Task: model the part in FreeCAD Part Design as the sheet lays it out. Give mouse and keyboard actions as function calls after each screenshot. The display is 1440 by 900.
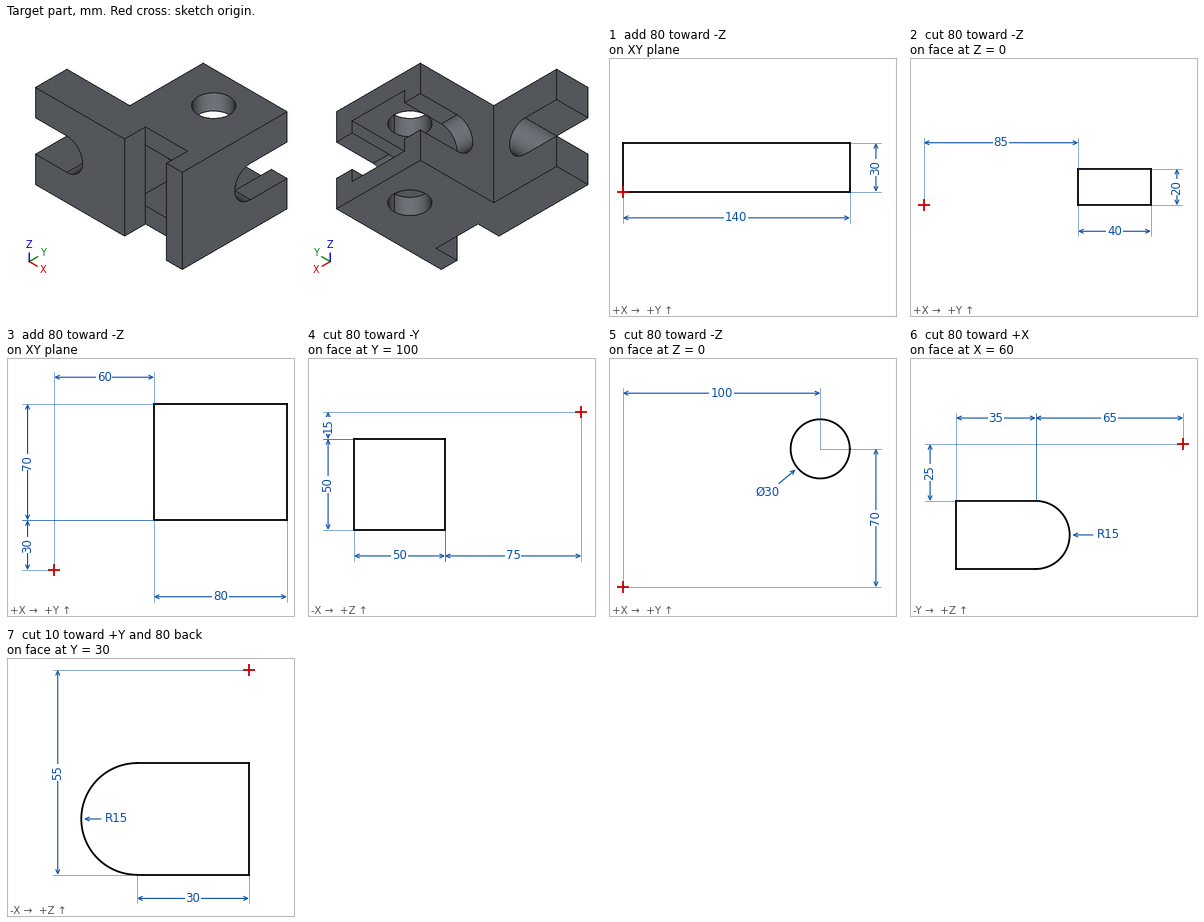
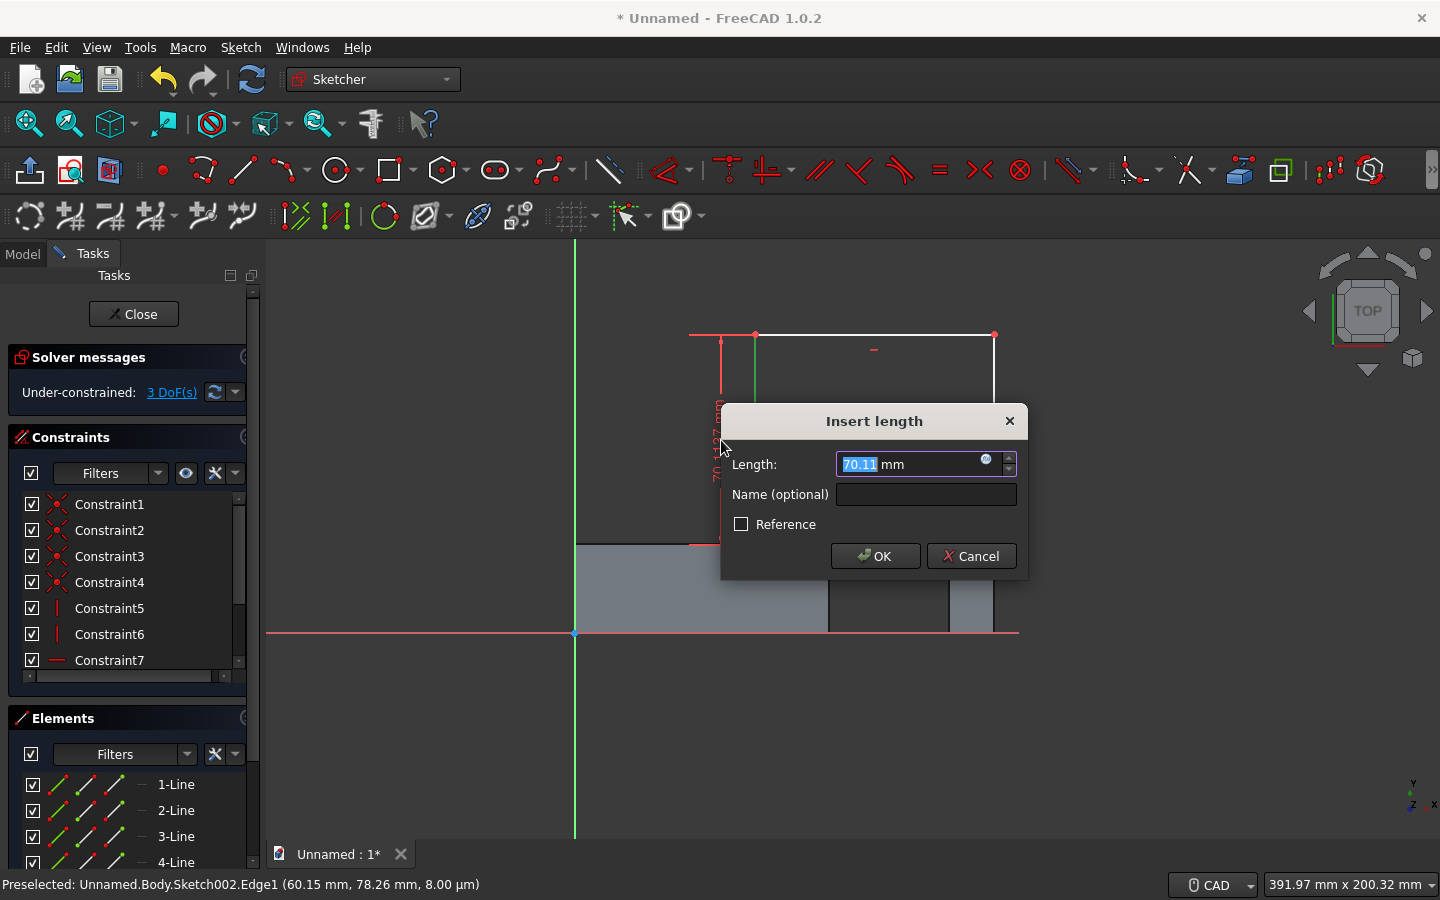
text(70)
key(Return)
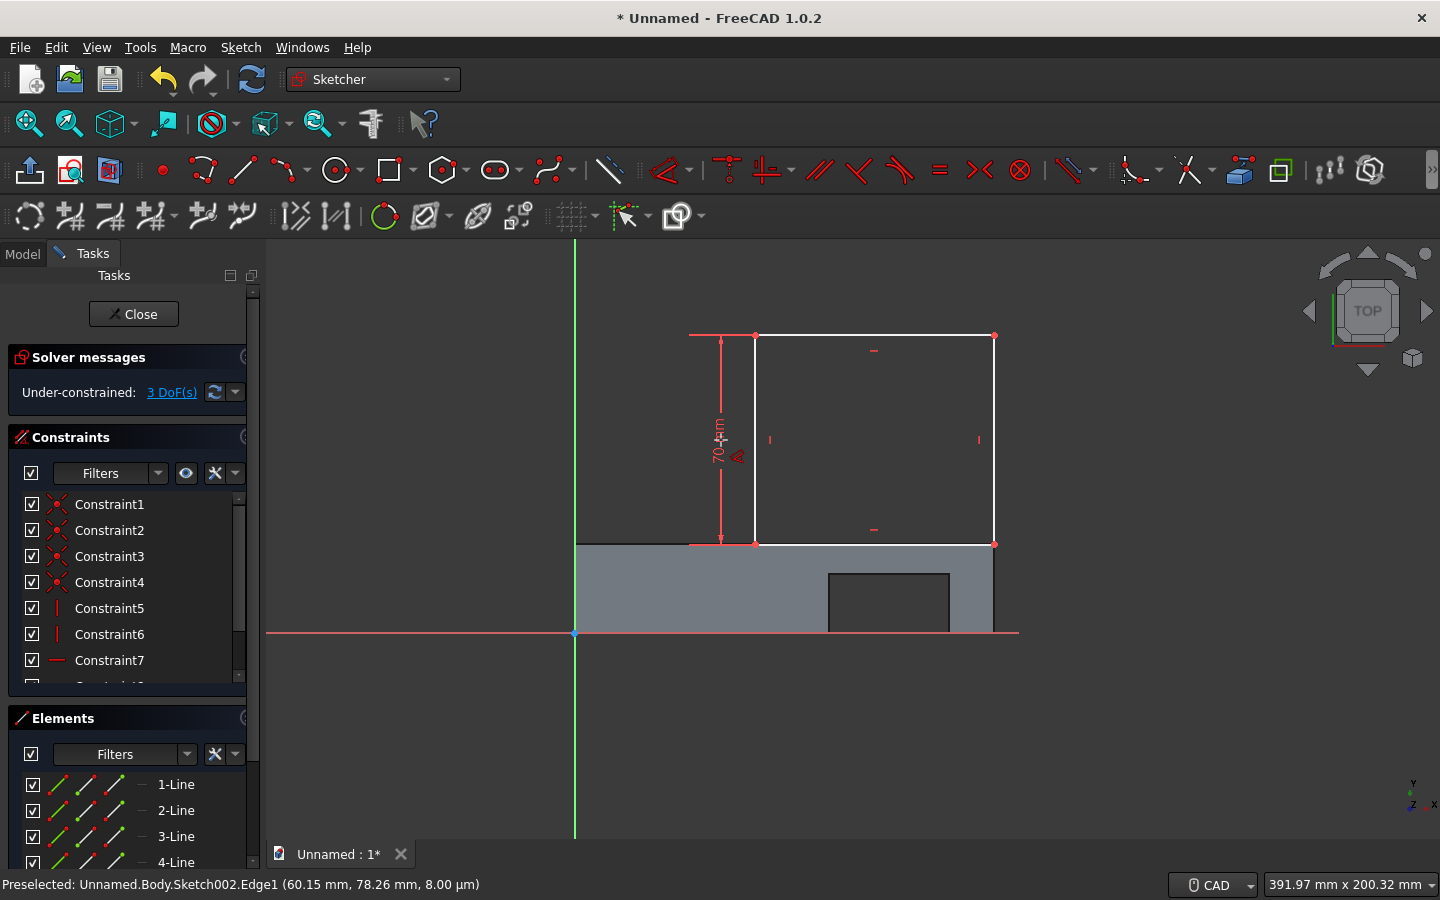
click(827, 545)
click(875, 579)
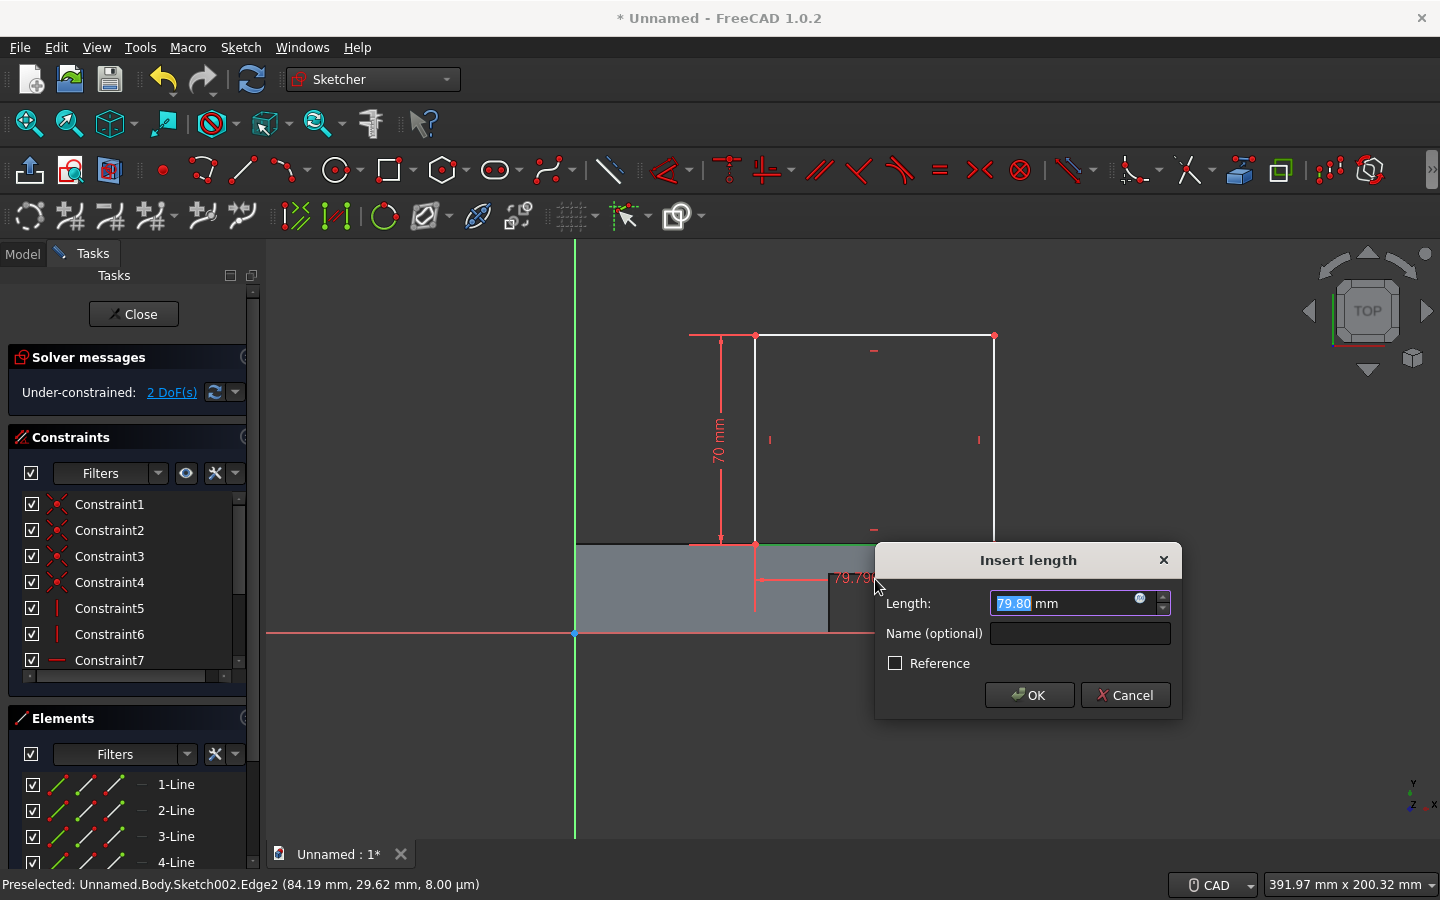
text(80)
key(Return)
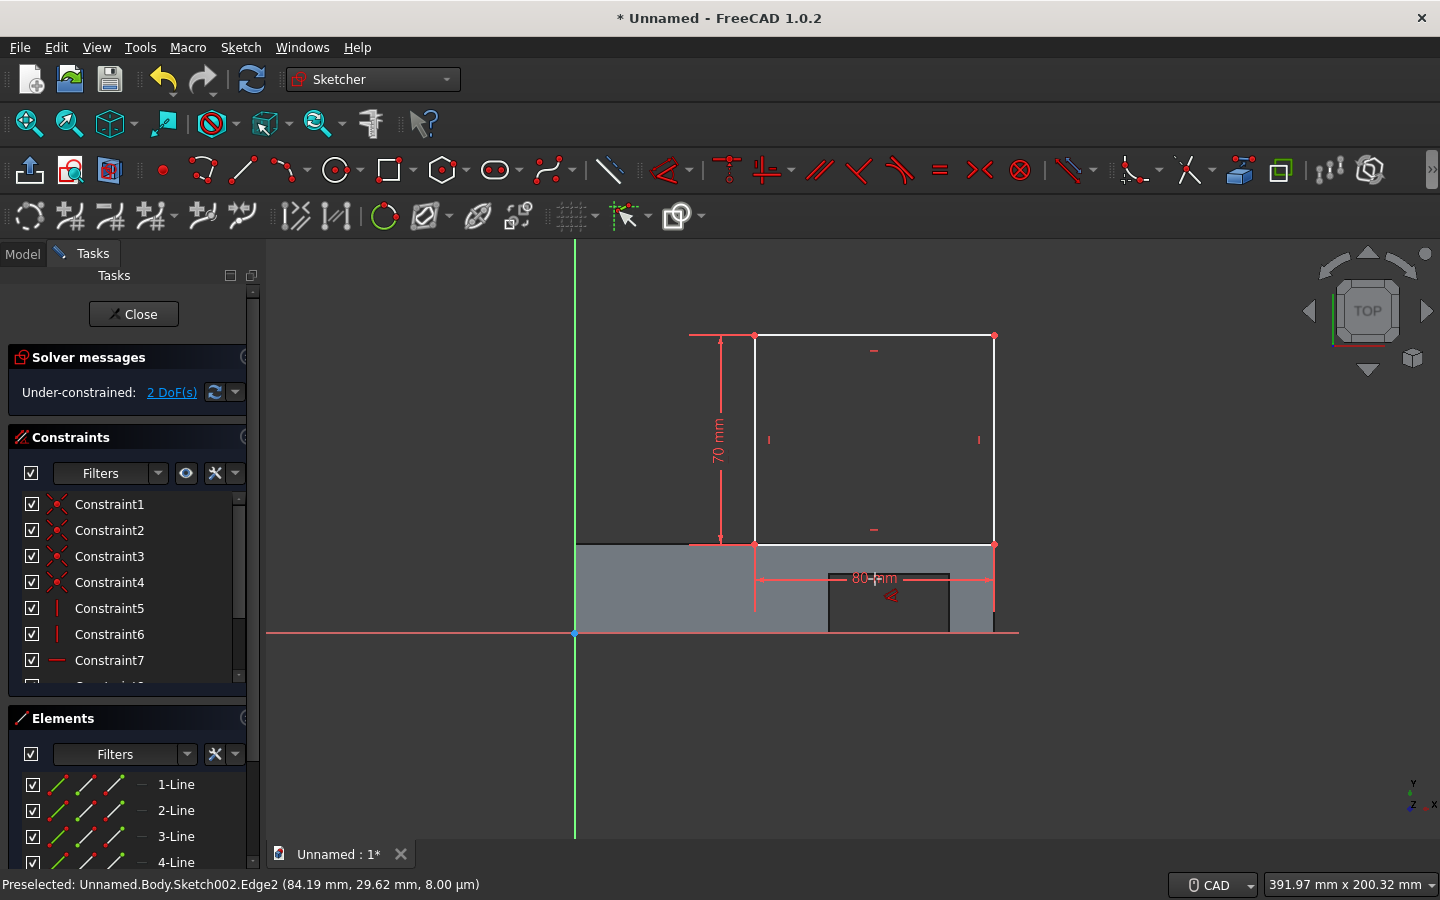
click(755, 335)
click(665, 667)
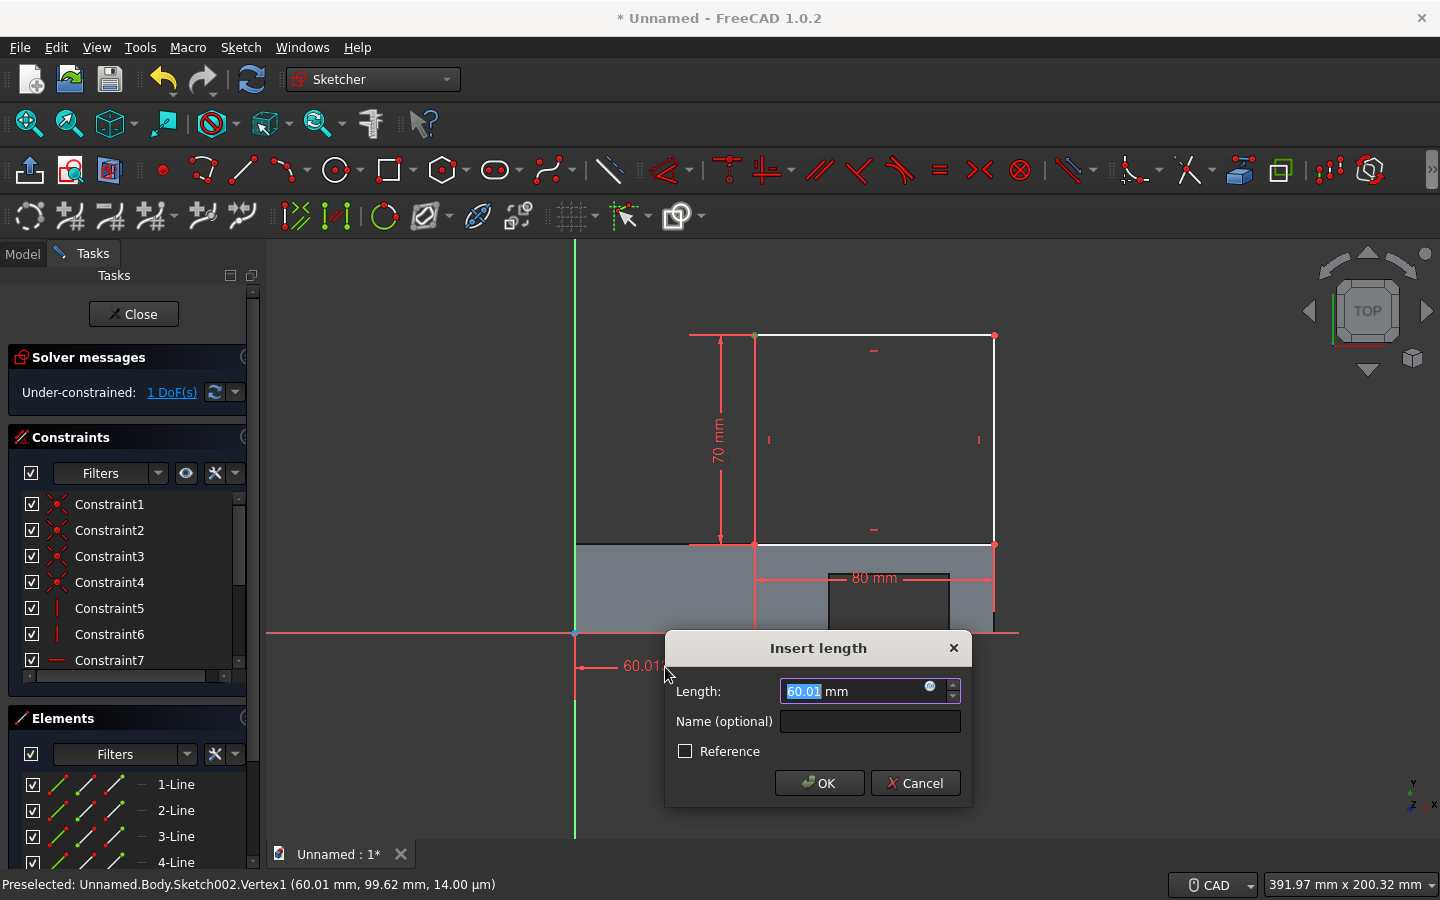
text(60)
key(Return)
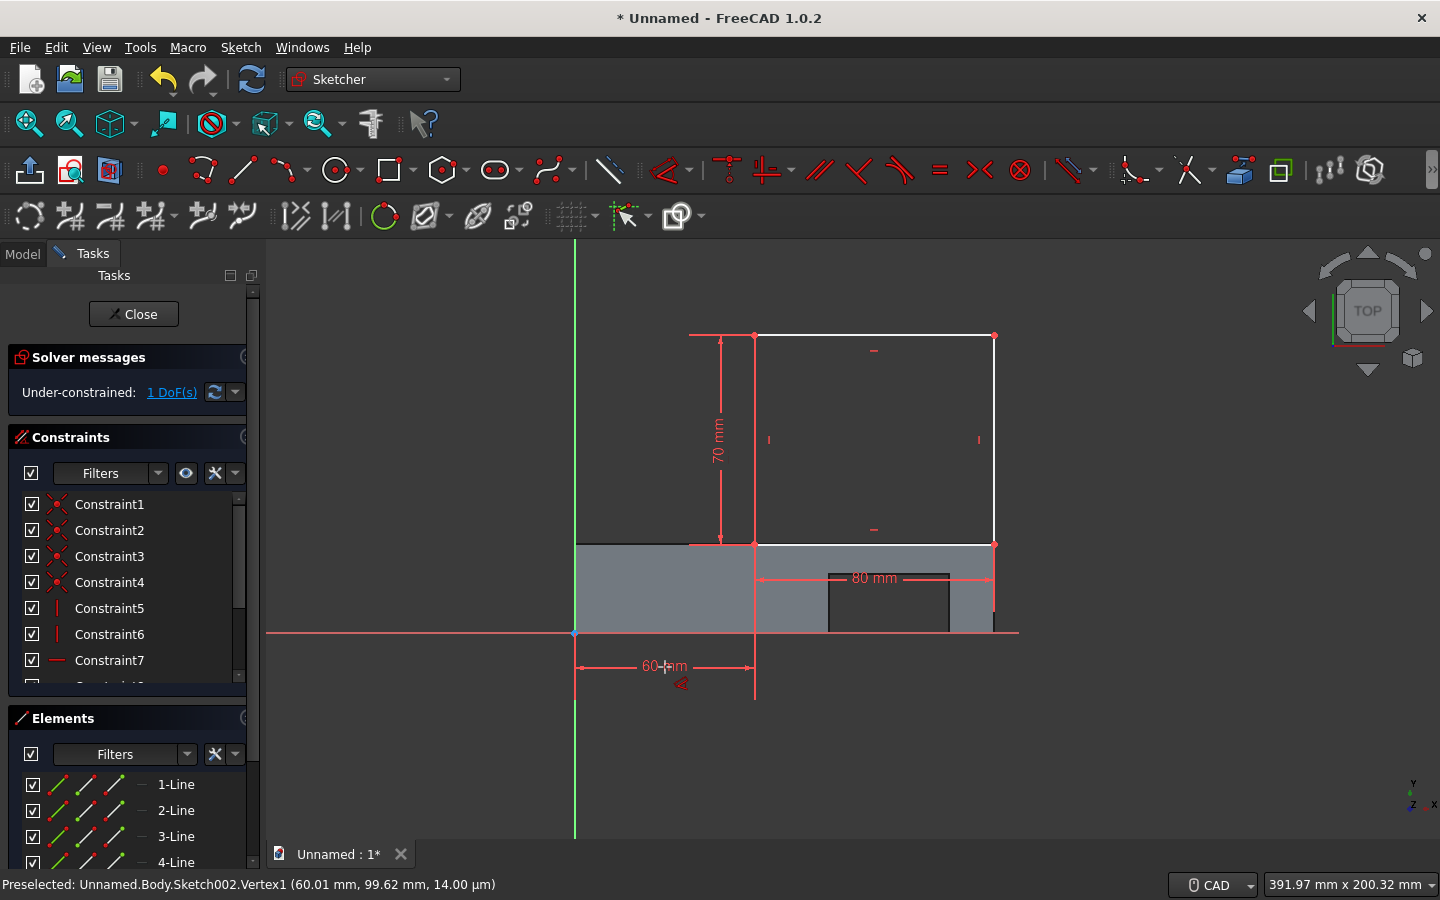
click(755, 545)
click(541, 589)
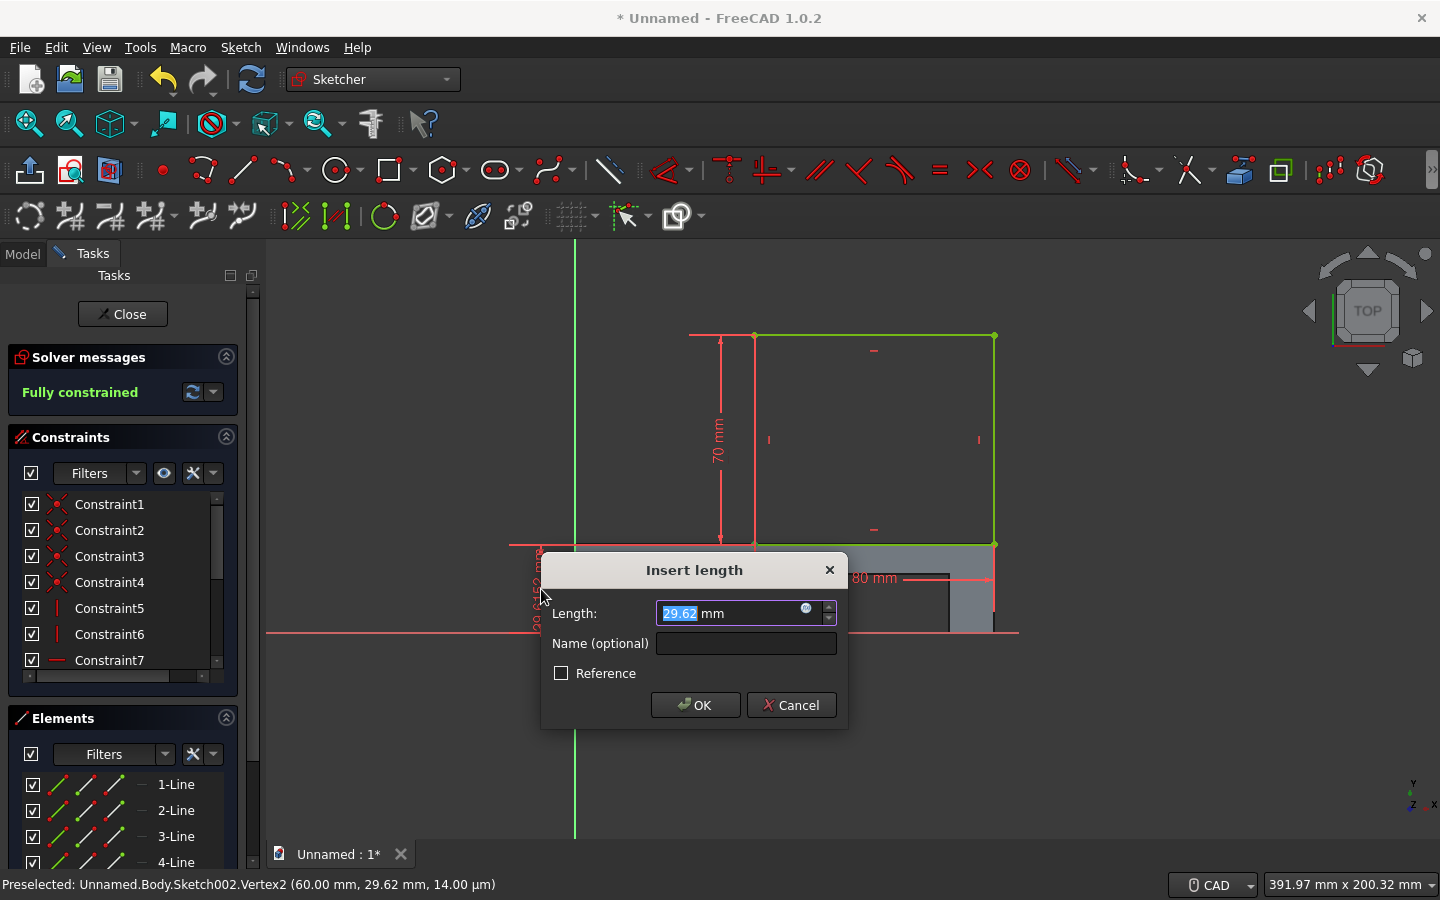
text(30)
key(Return)
key(Escape)